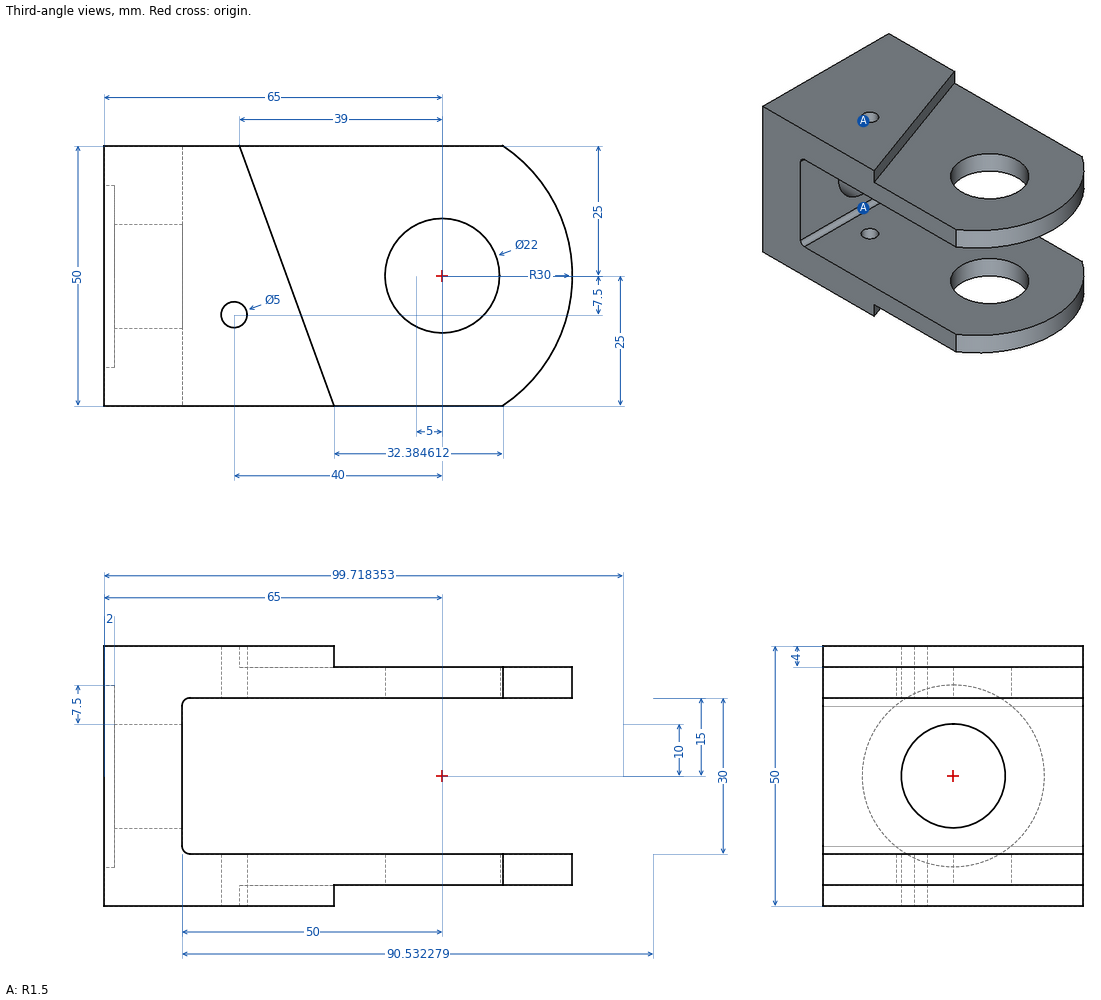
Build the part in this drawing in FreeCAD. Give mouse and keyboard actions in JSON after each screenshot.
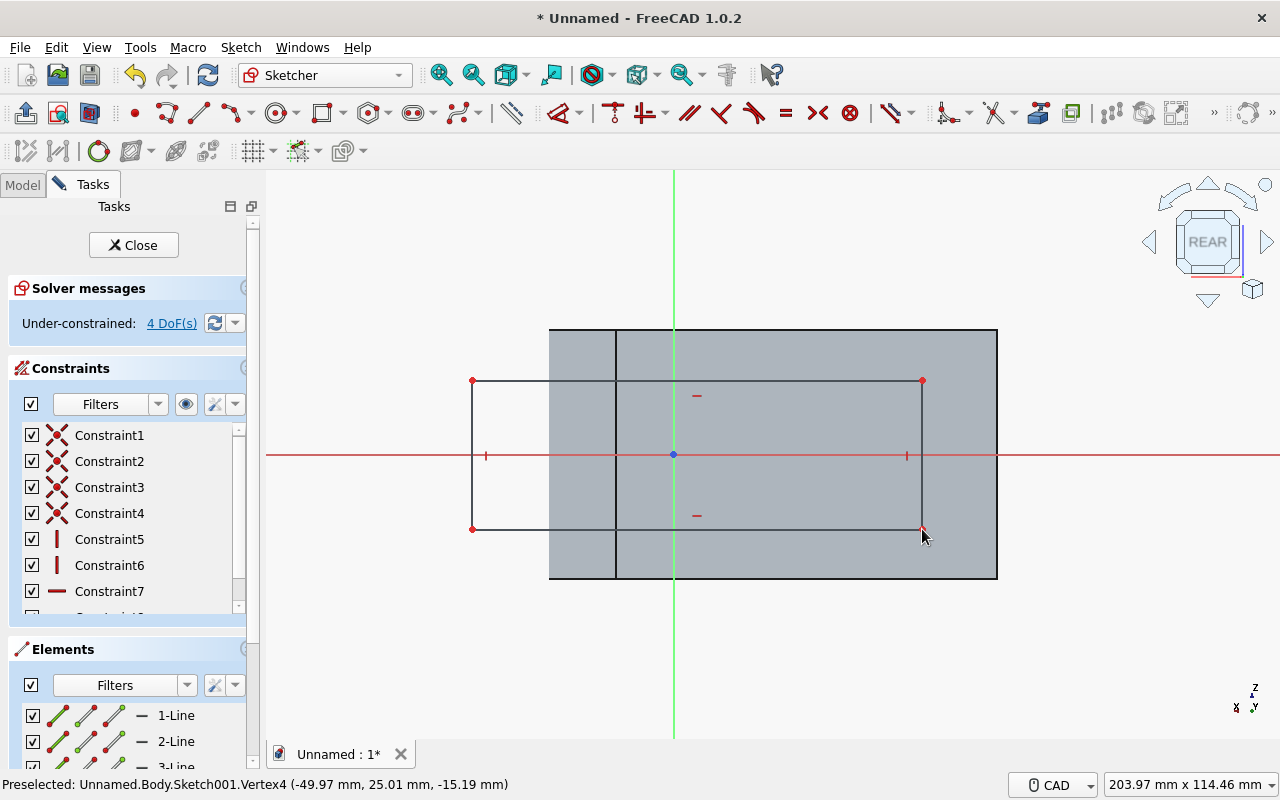
{"action": "left_click", "coordinate": [558, 114]}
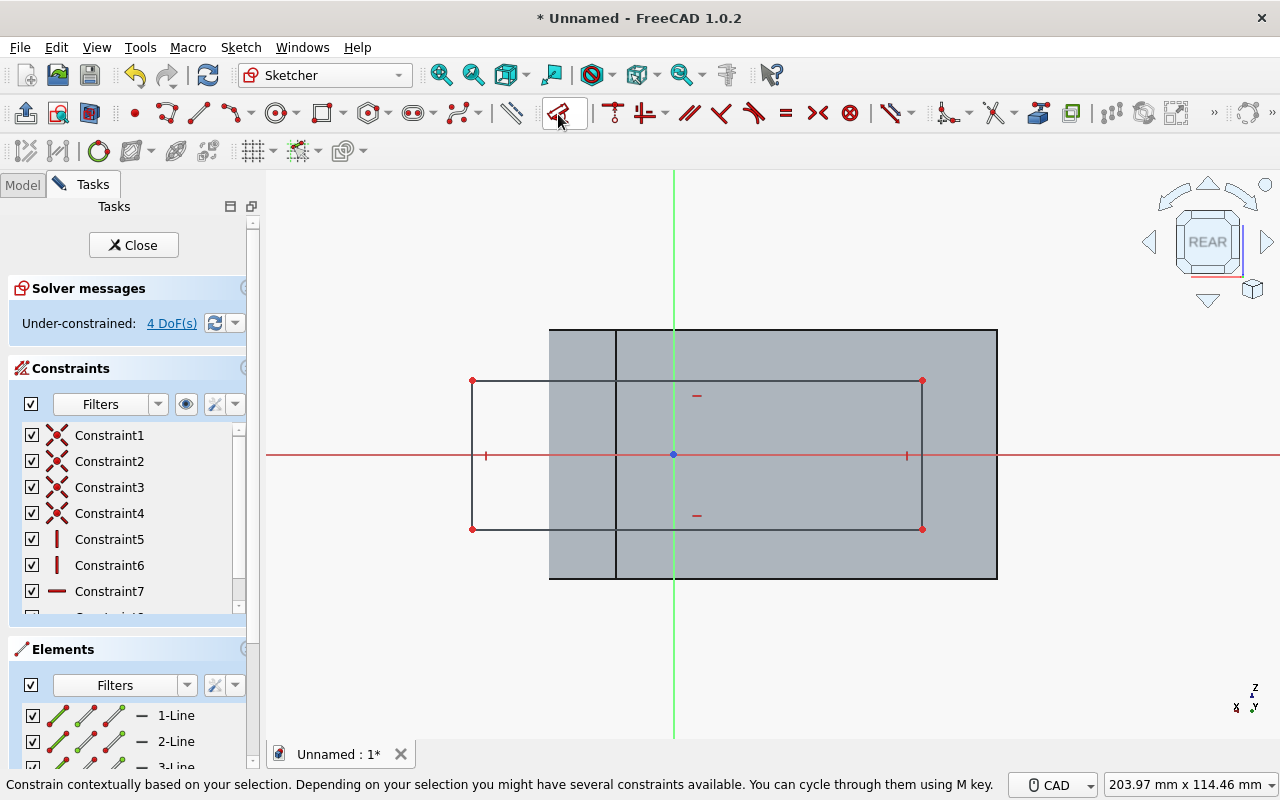
{"action": "left_click", "coordinate": [472, 426]}
{"action": "left_click", "coordinate": [438, 421]}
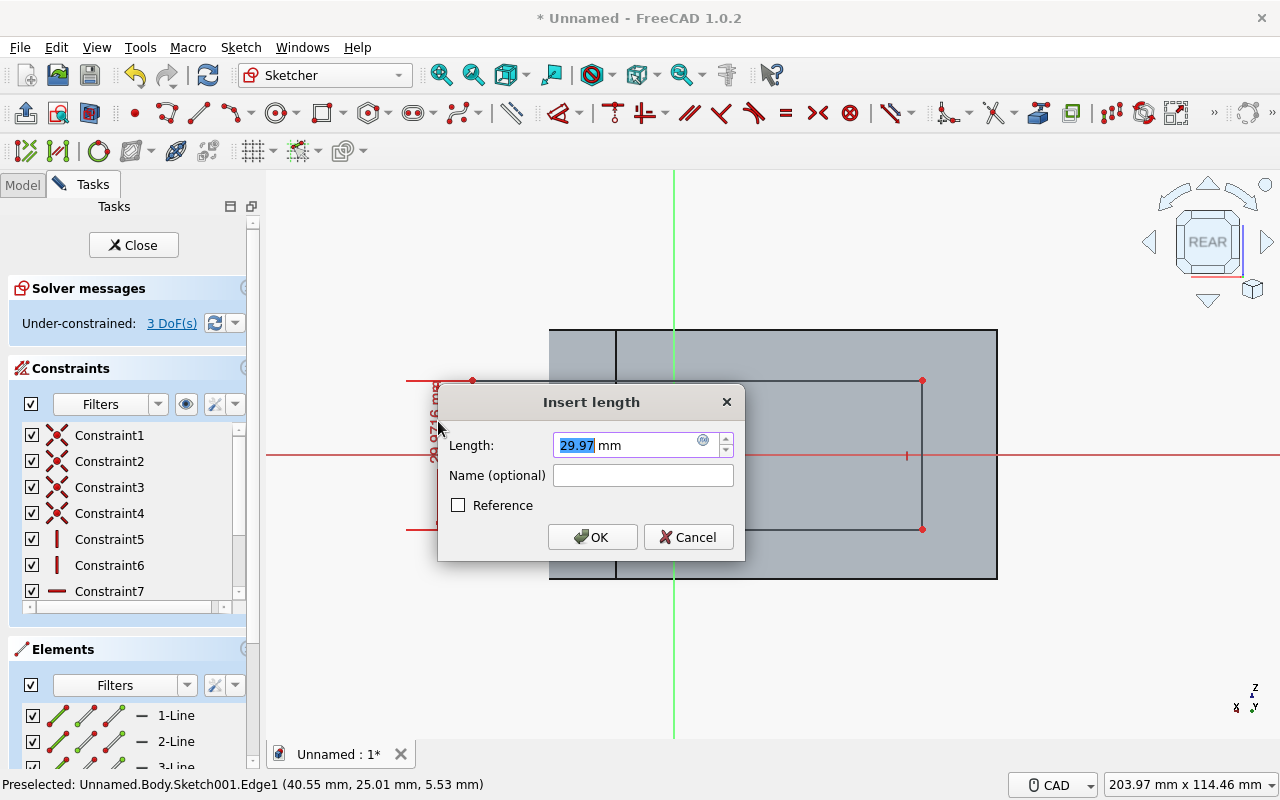
{"action": "type", "text": "30"}
{"action": "key", "text": "Return"}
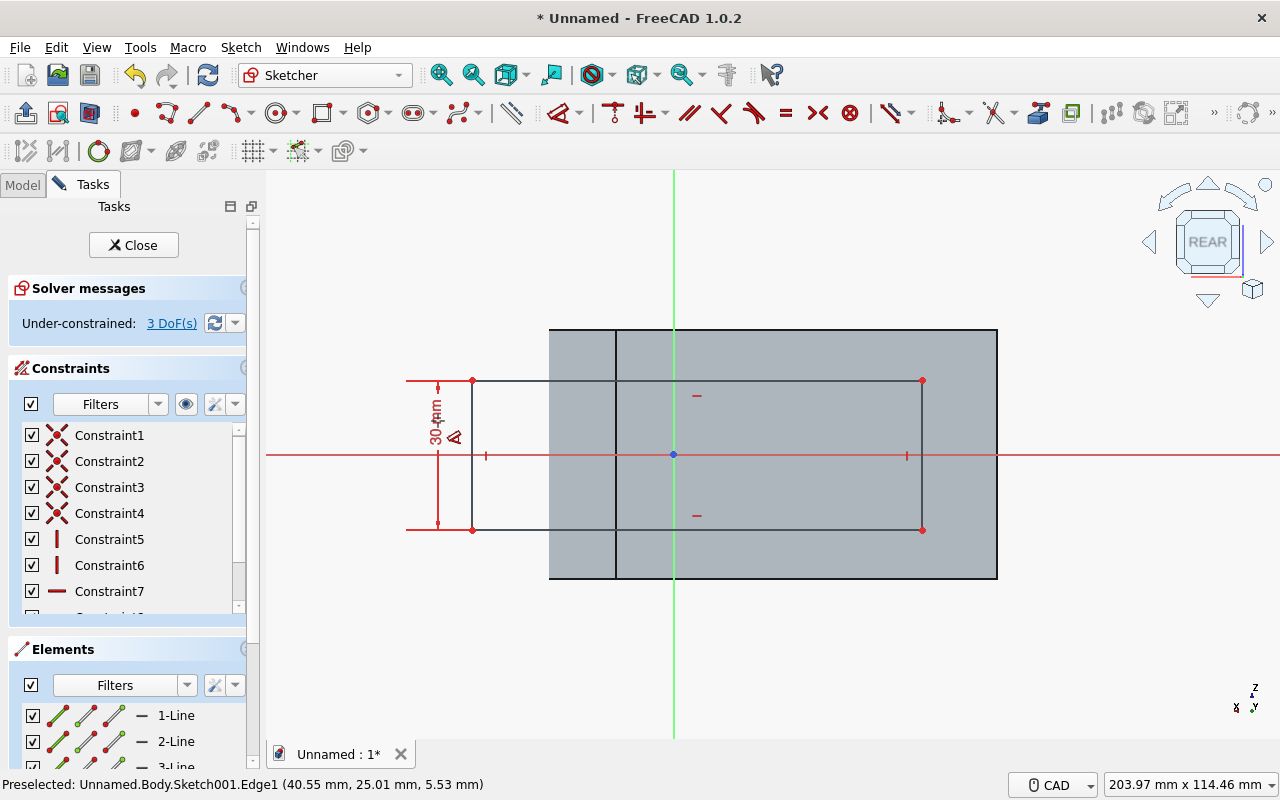
{"action": "left_click", "coordinate": [472, 381]}
{"action": "left_click", "coordinate": [438, 401]}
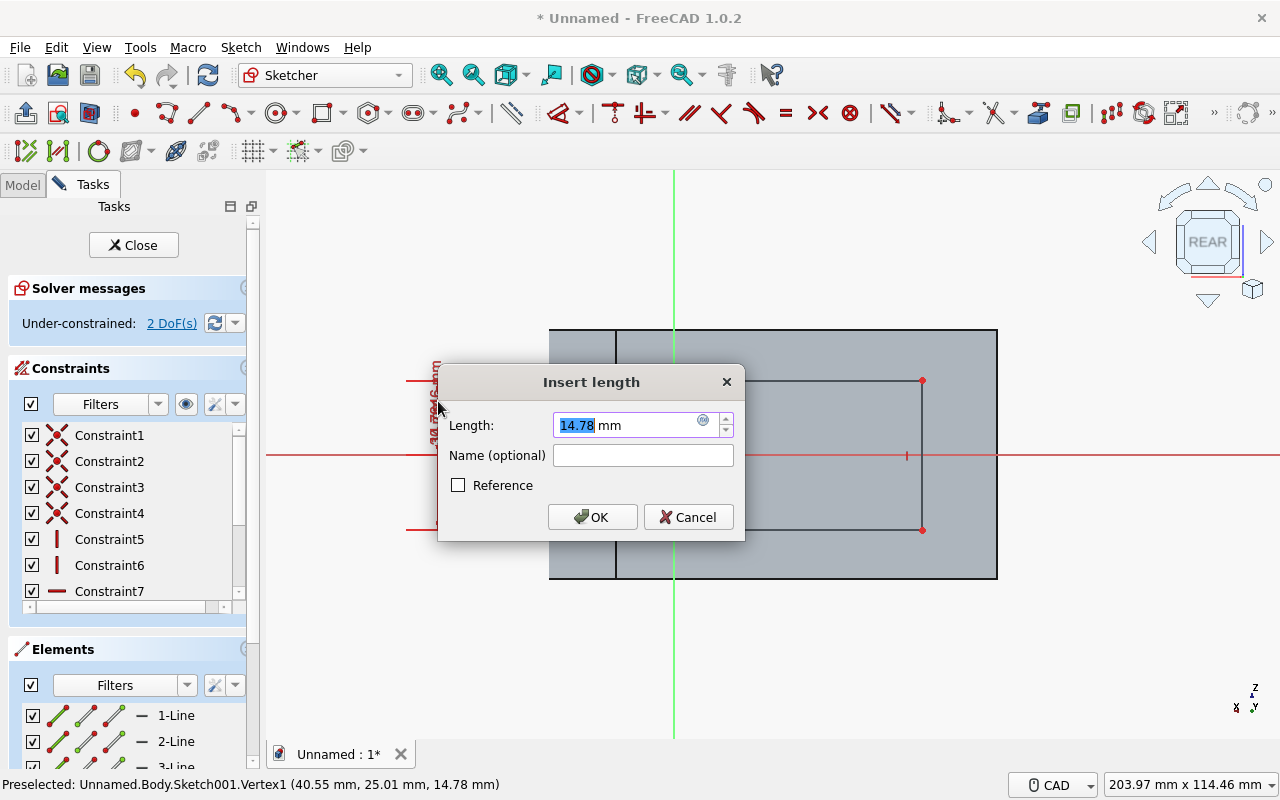
{"action": "type", "text": "15"}
{"action": "key", "text": "Return"}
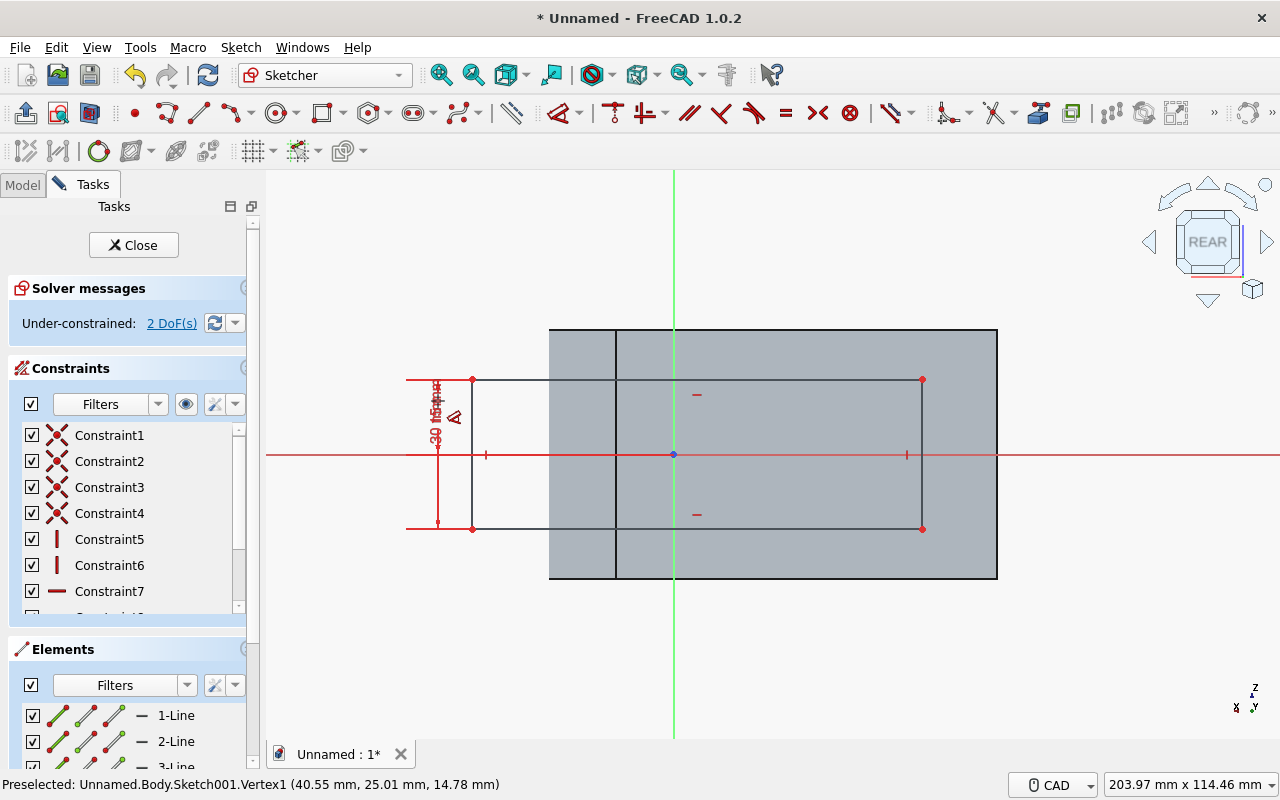
{"action": "left_click", "coordinate": [922, 529]}
{"action": "left_click", "coordinate": [798, 563]}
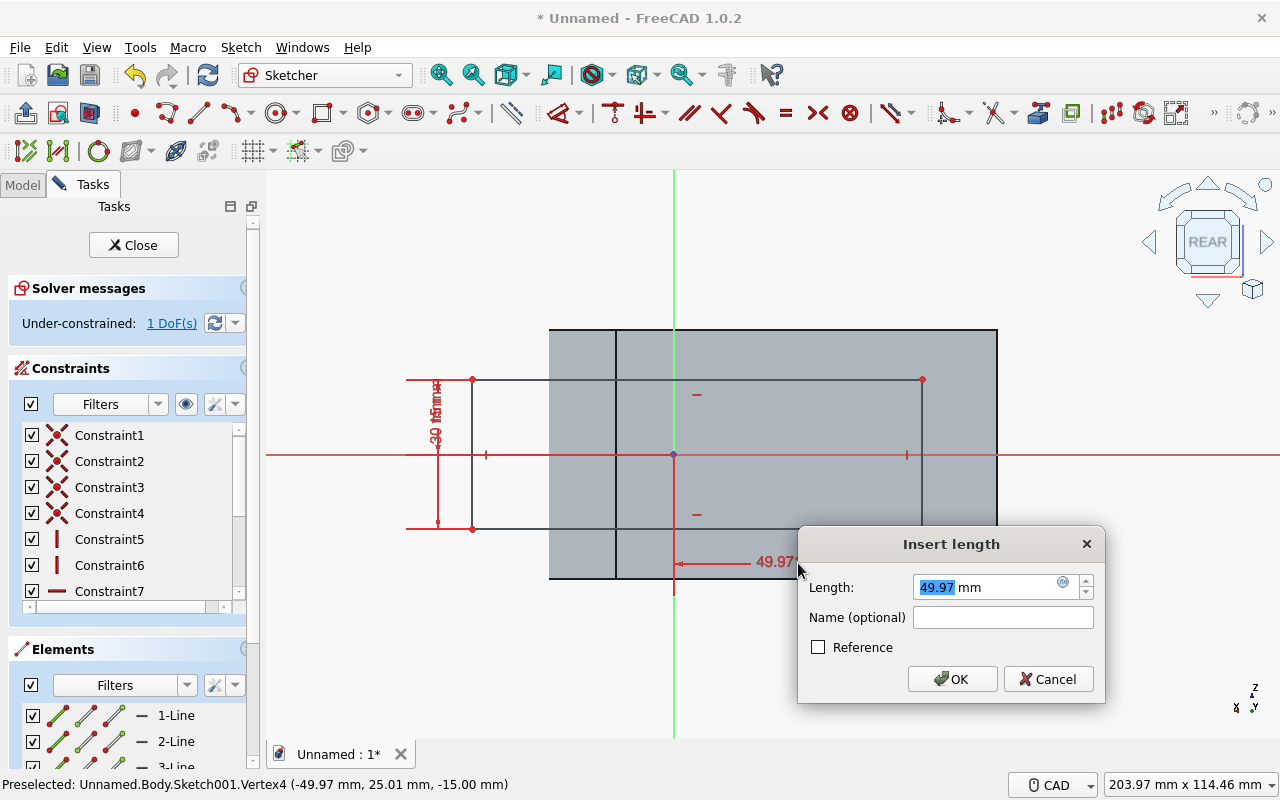
{"action": "type", "text": "50"}
{"action": "key", "text": "Return"}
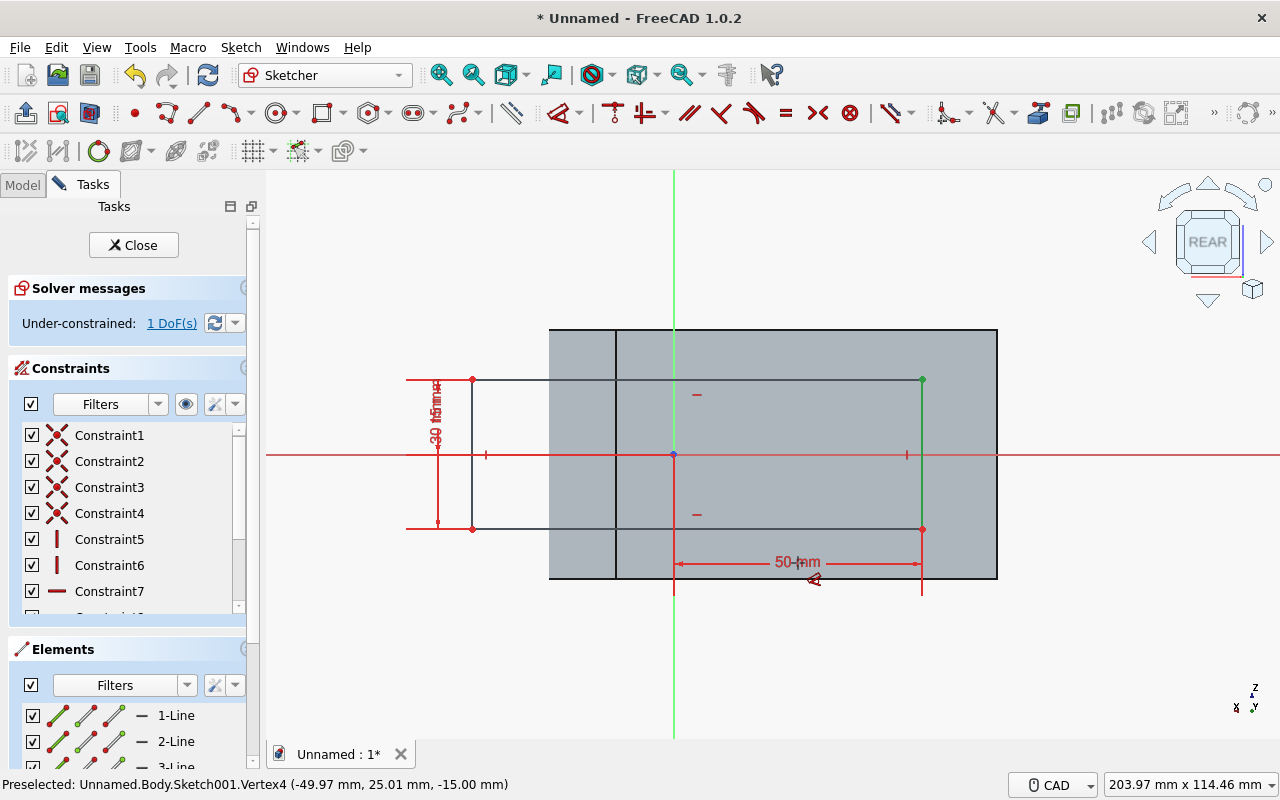
{"action": "left_click", "coordinate": [607, 529]}
{"action": "left_click", "coordinate": [697, 563]}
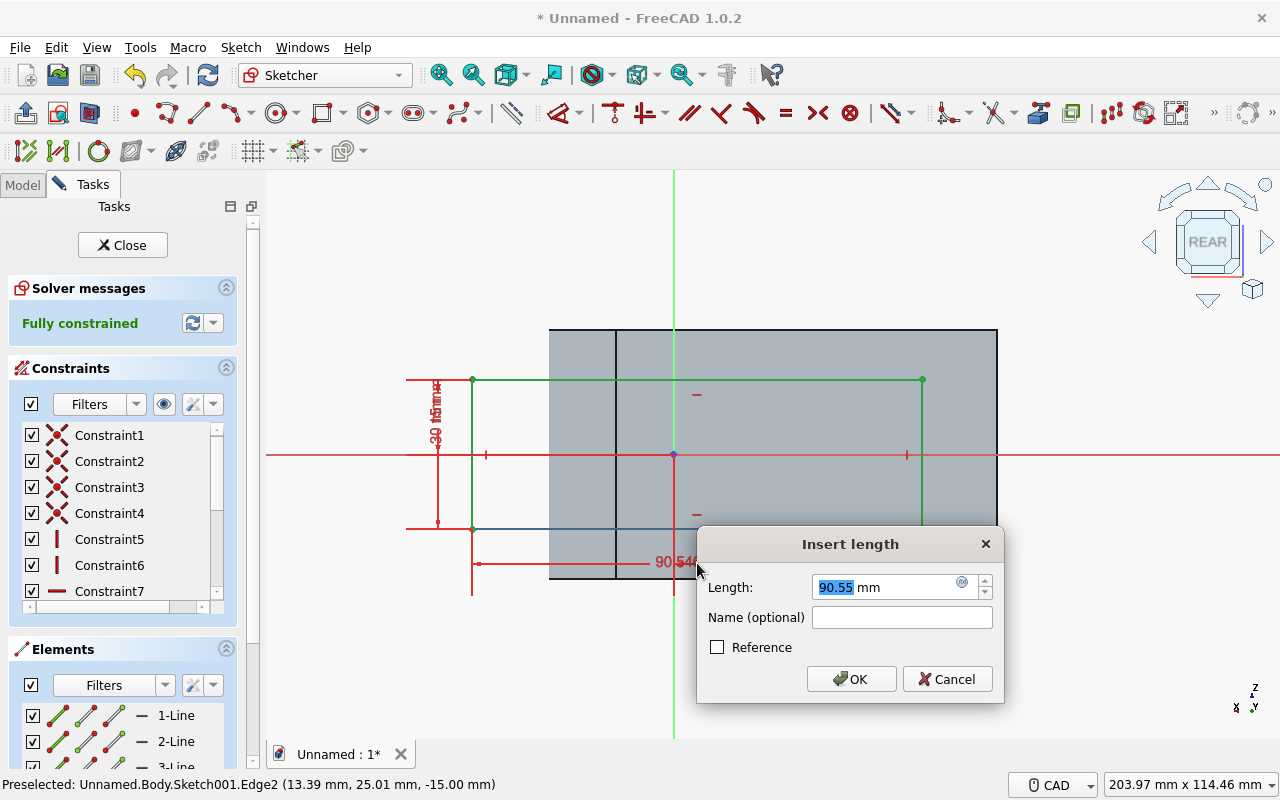
{"action": "type", "text": "90.532279"}
{"action": "key", "text": "Return"}
{"action": "key", "text": "Escape"}